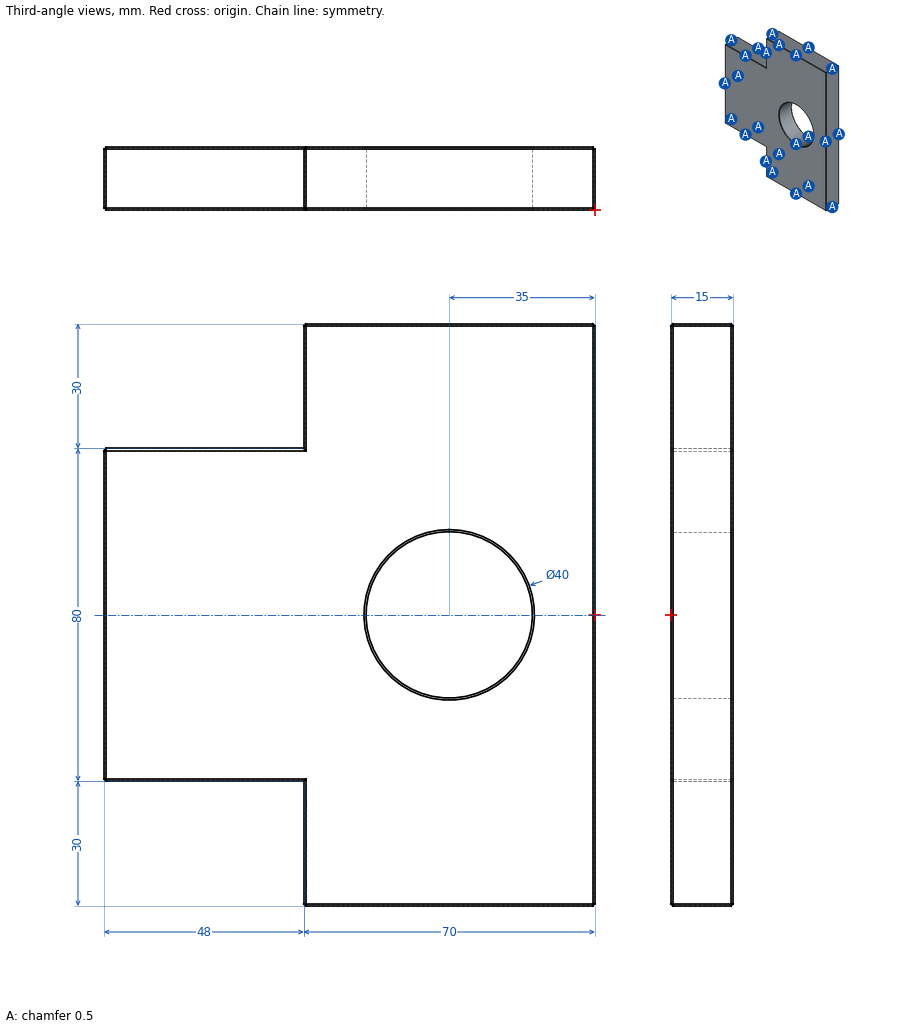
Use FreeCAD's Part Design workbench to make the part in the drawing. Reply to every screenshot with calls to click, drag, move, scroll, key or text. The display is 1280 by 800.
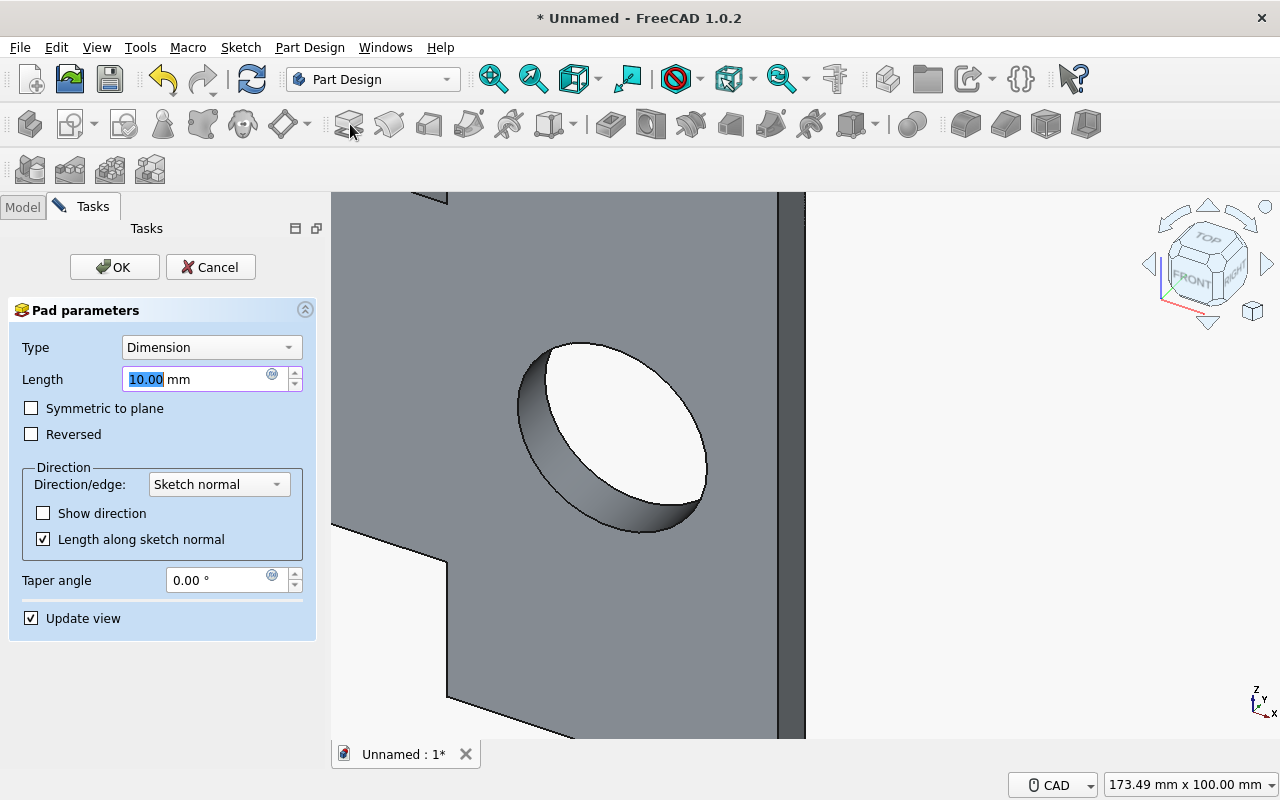
text(15)
key(Tab)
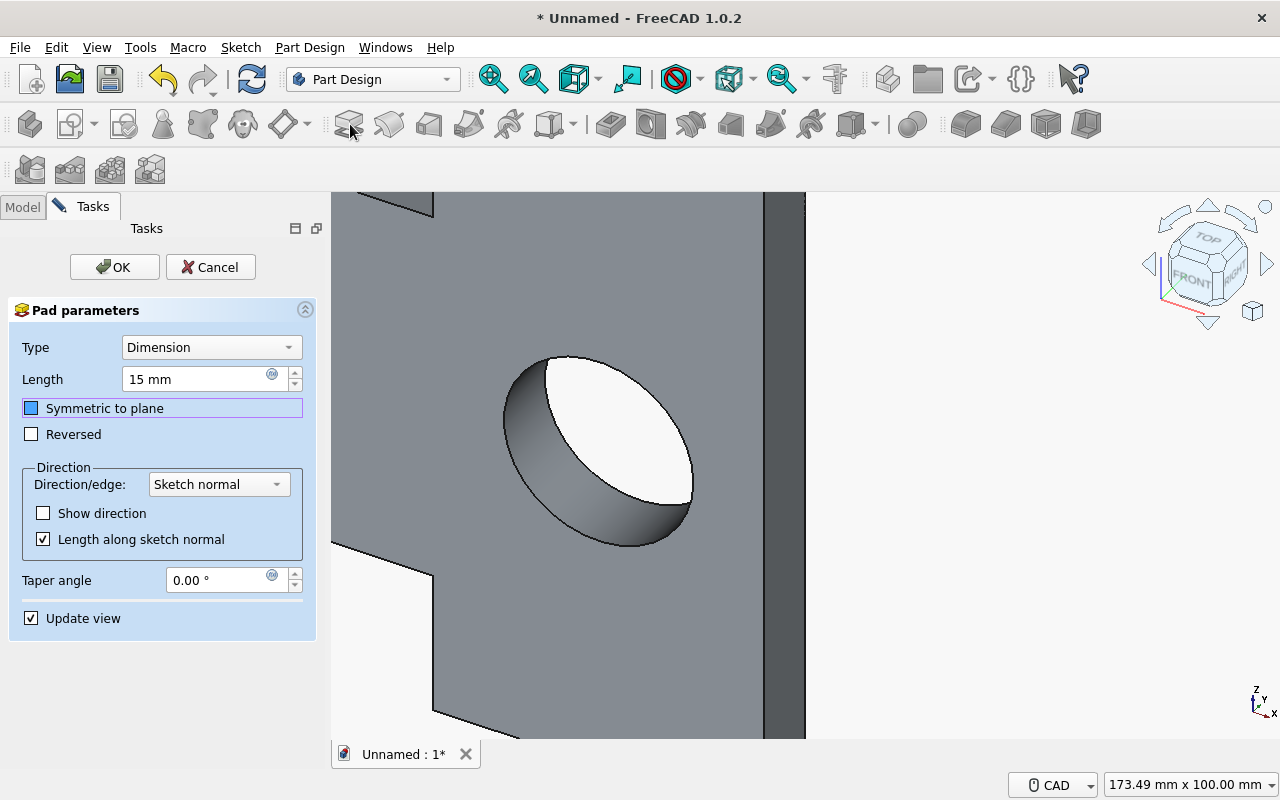
click(30, 434)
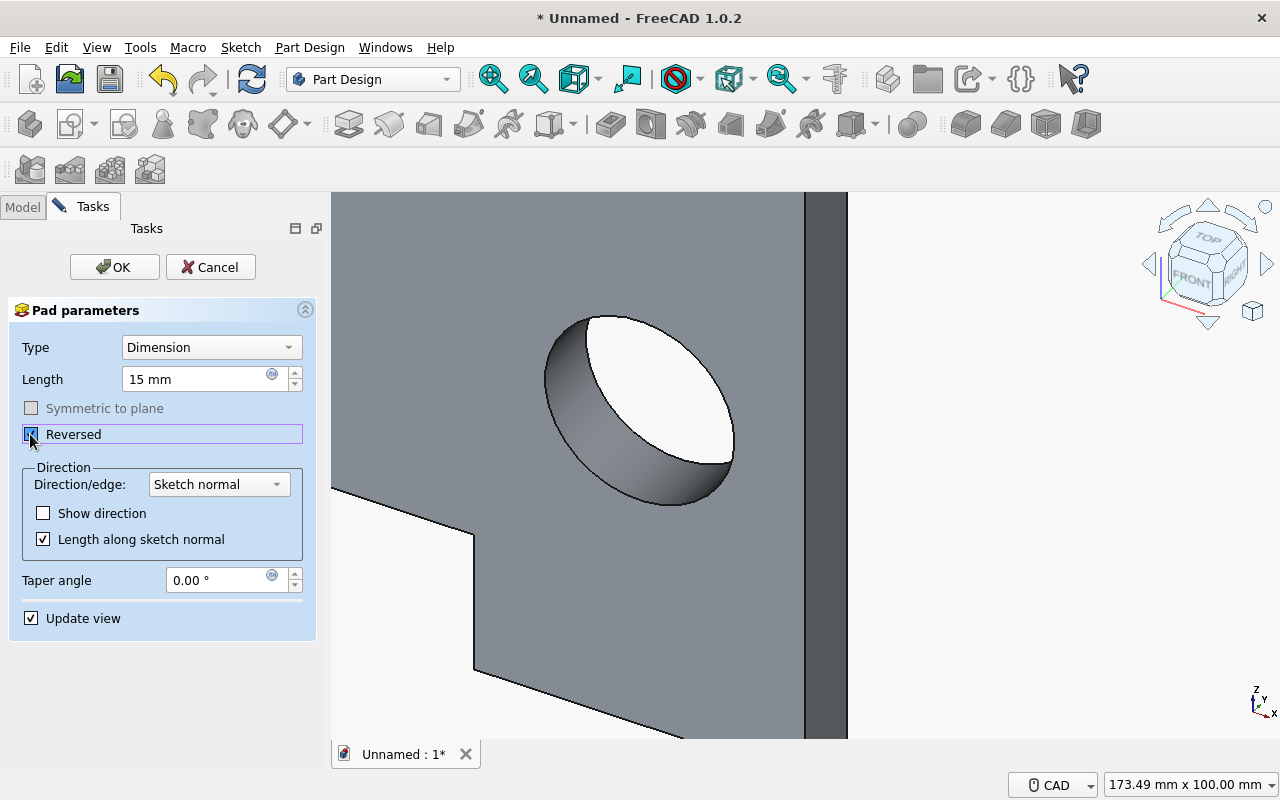
click(115, 267)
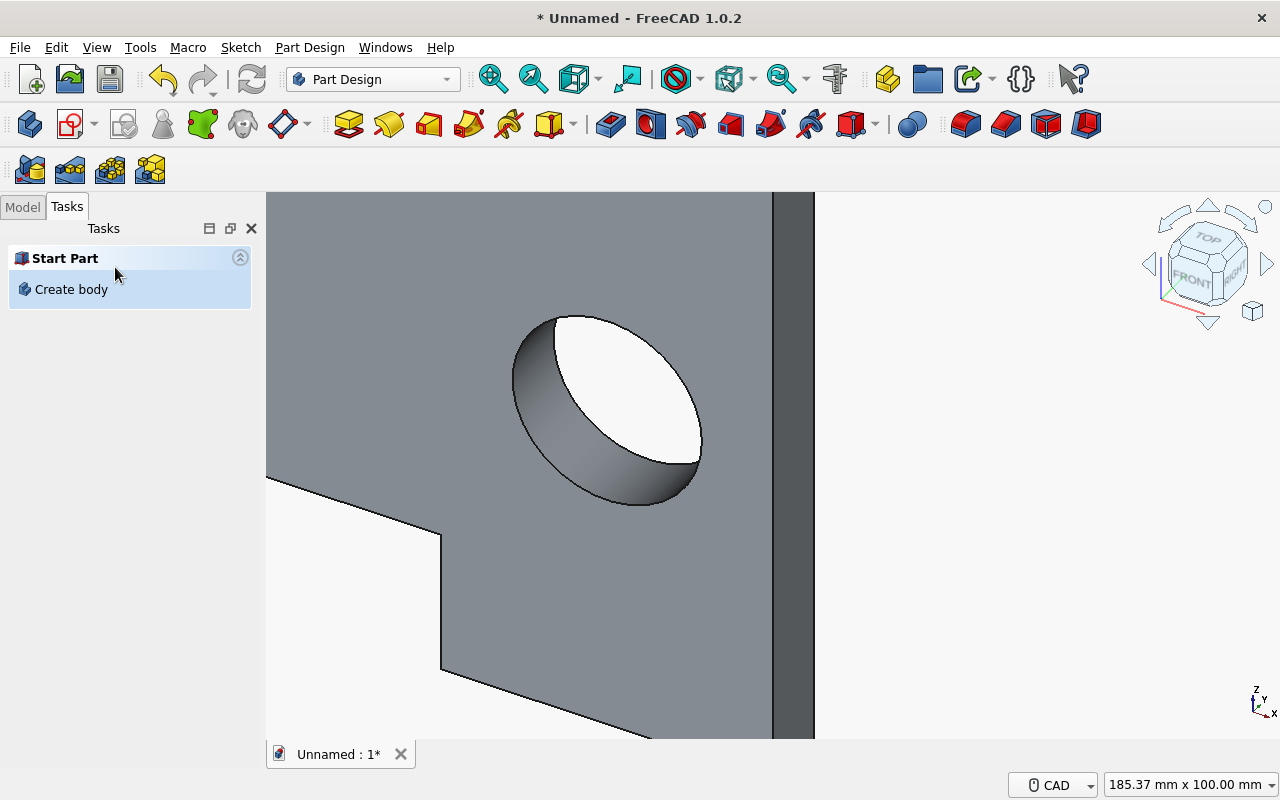
click(494, 80)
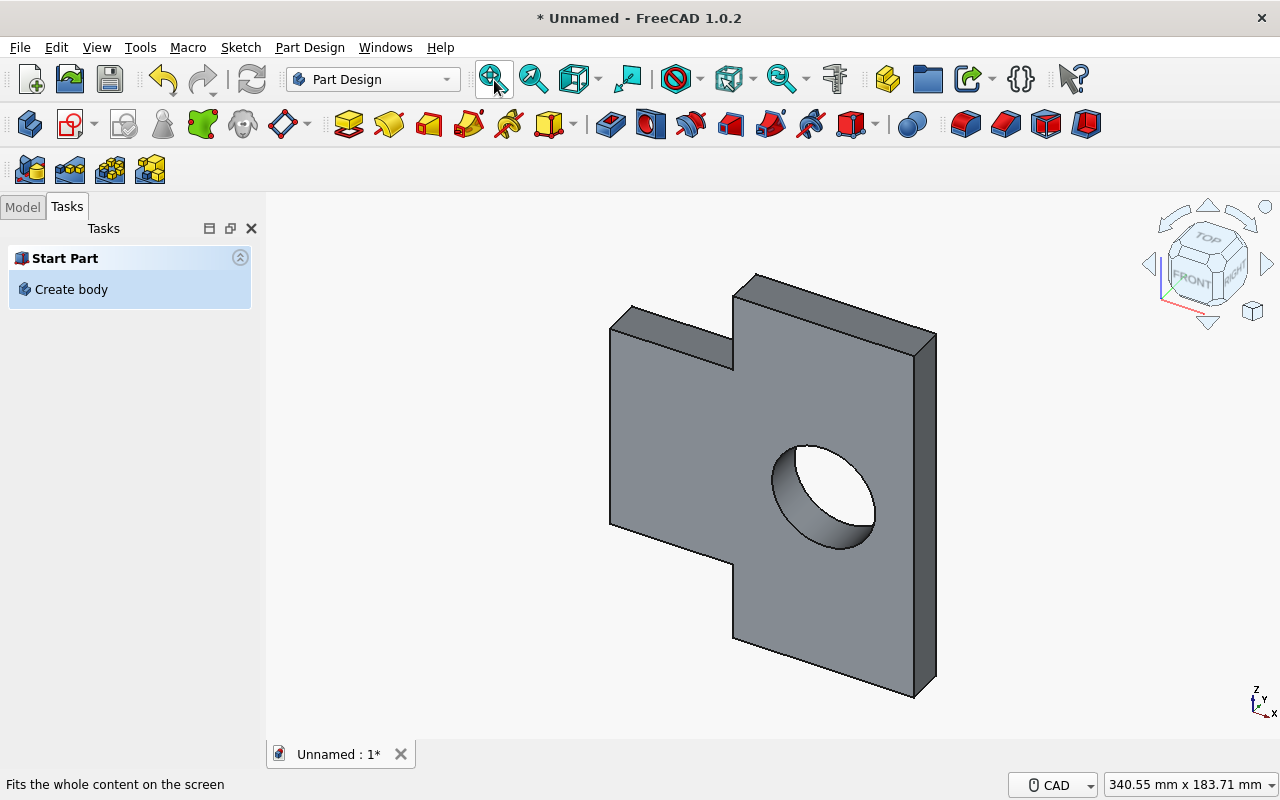
click(675, 447)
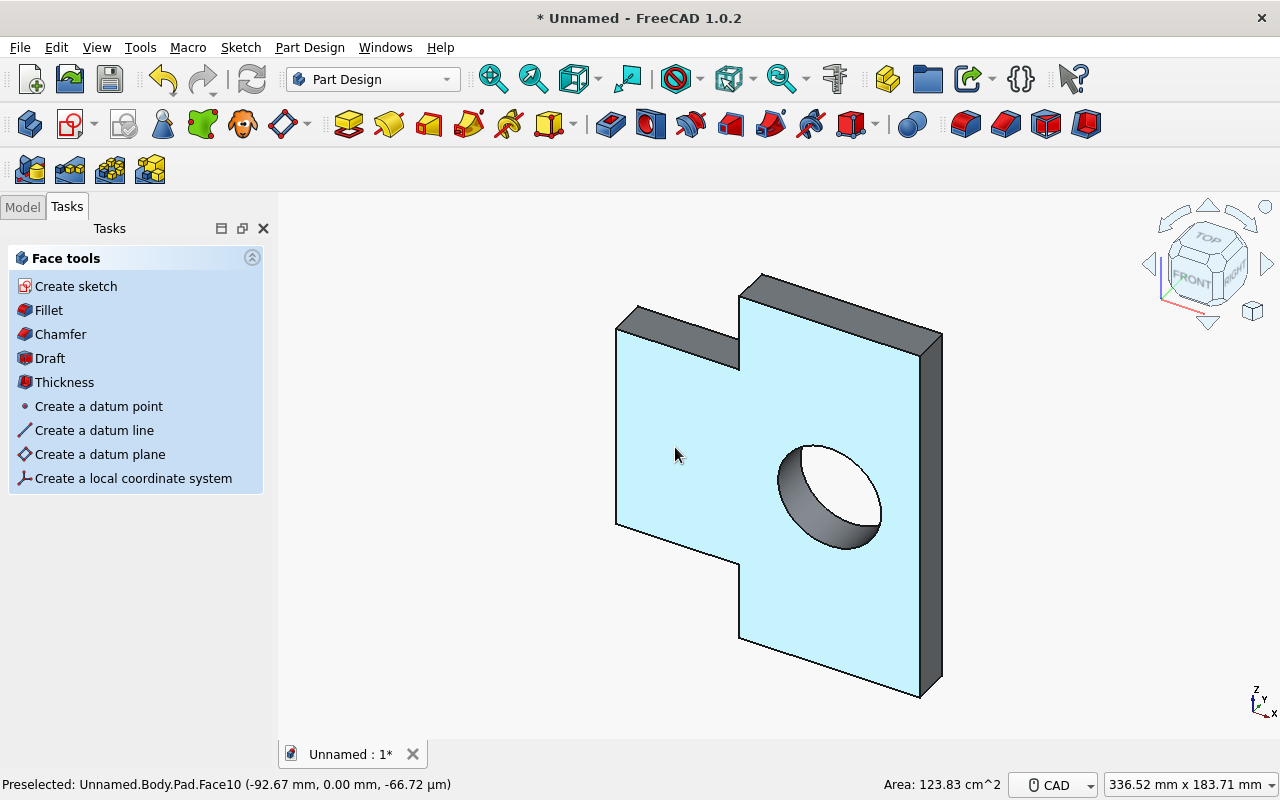
click(931, 344, ctrl)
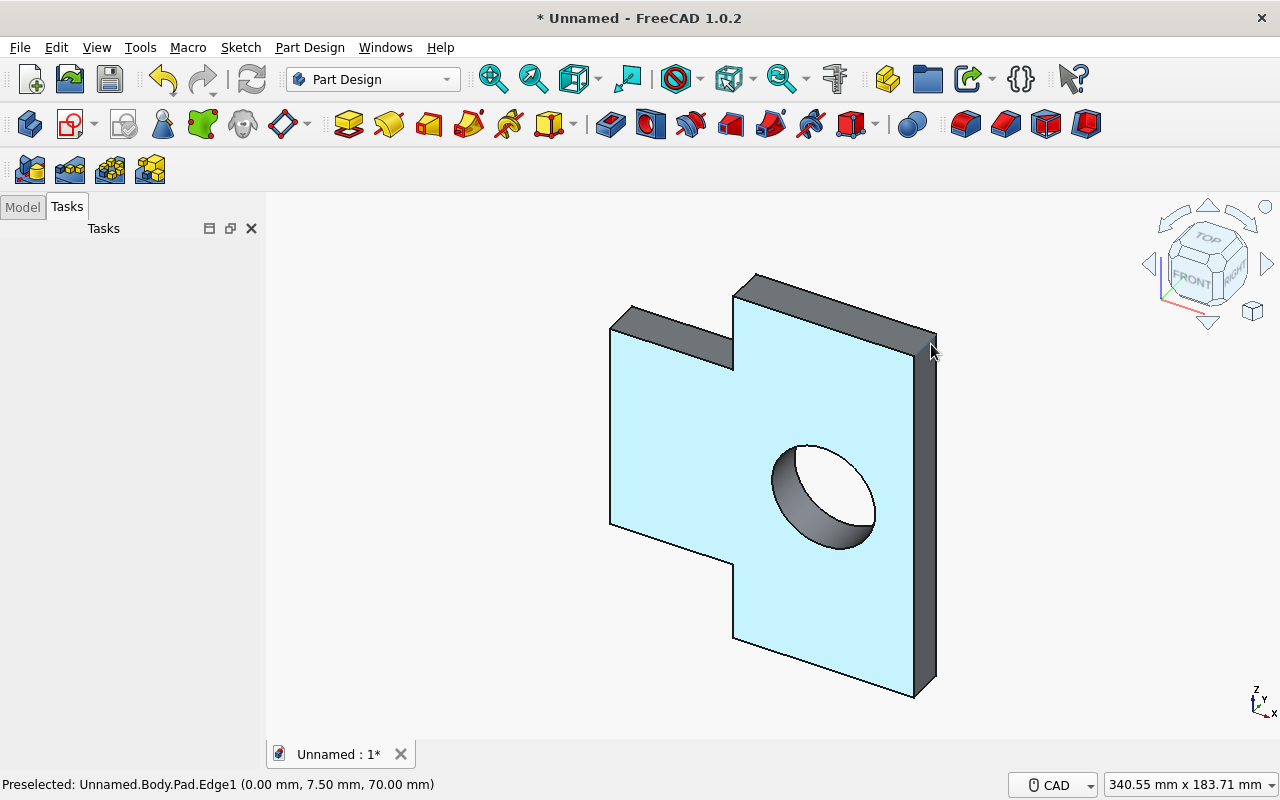
key(0)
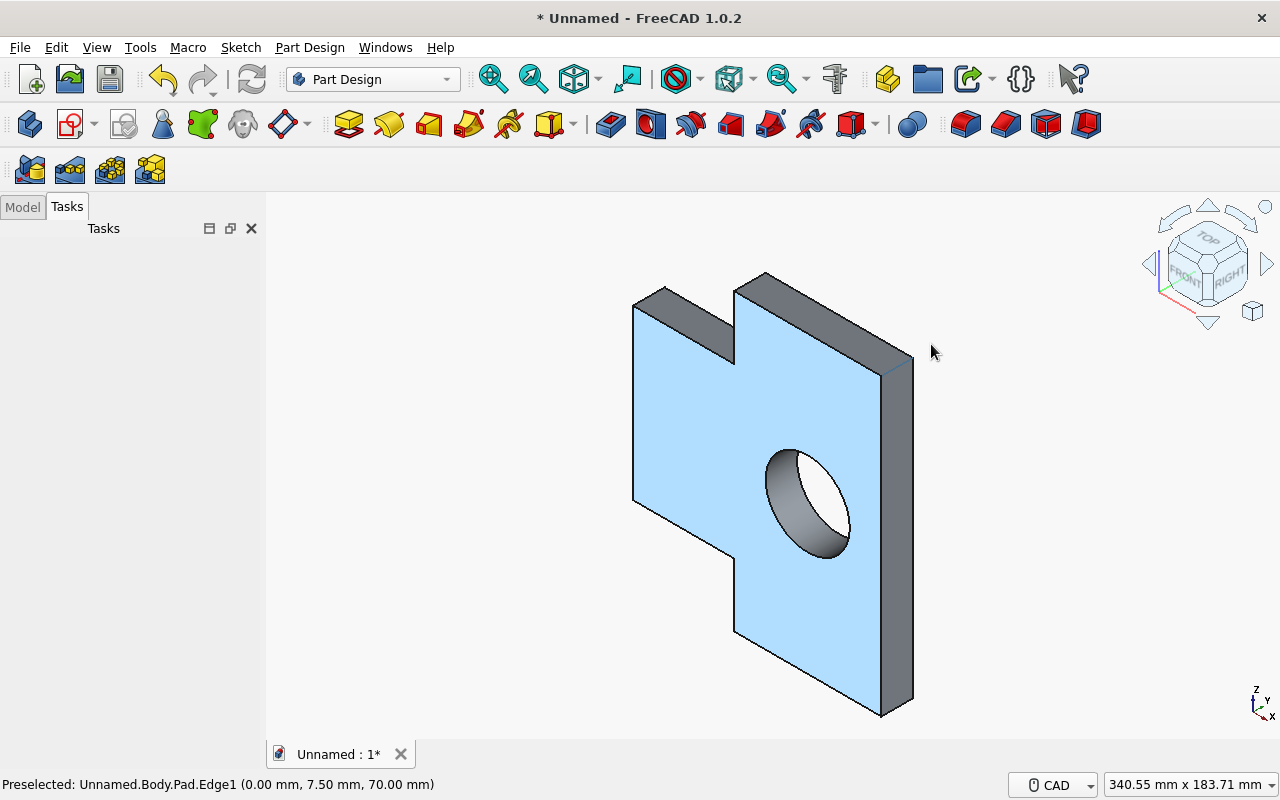
key(2)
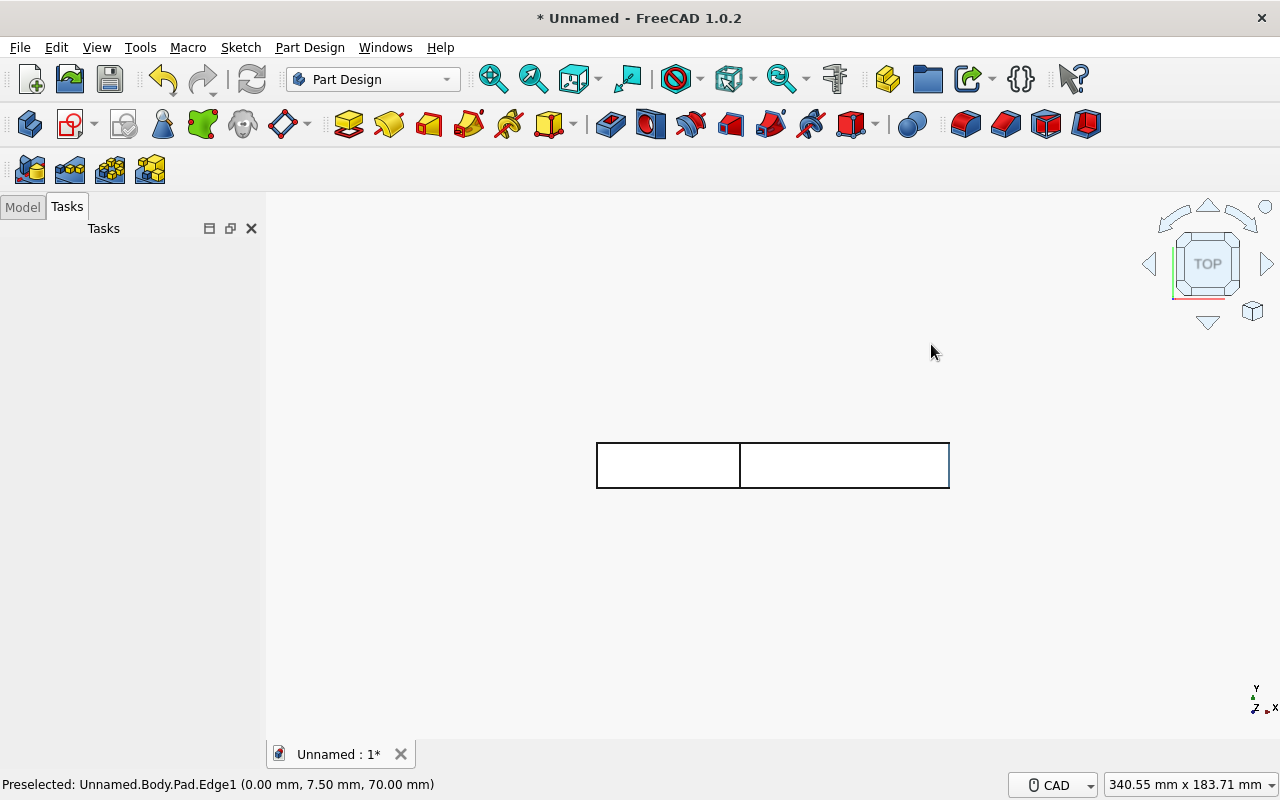
key(v)
key(f)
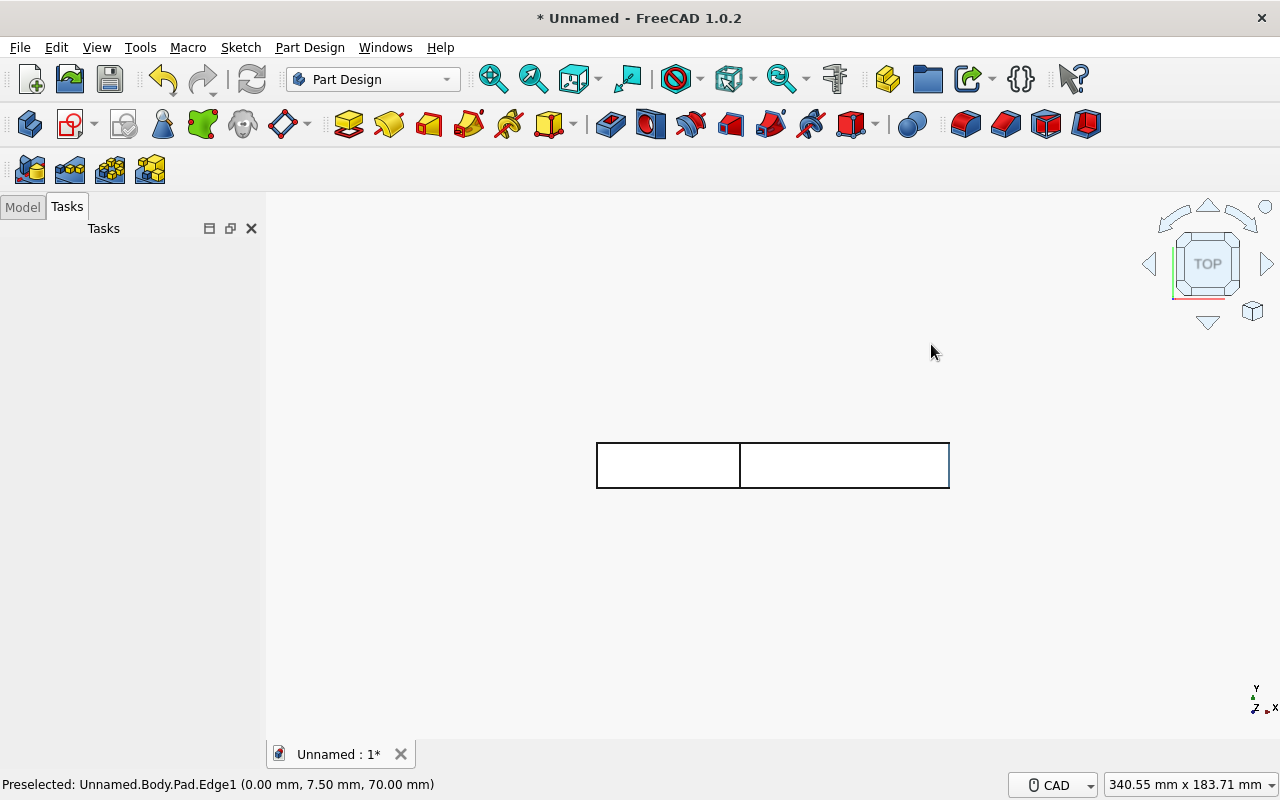
click(740, 464, ctrl)